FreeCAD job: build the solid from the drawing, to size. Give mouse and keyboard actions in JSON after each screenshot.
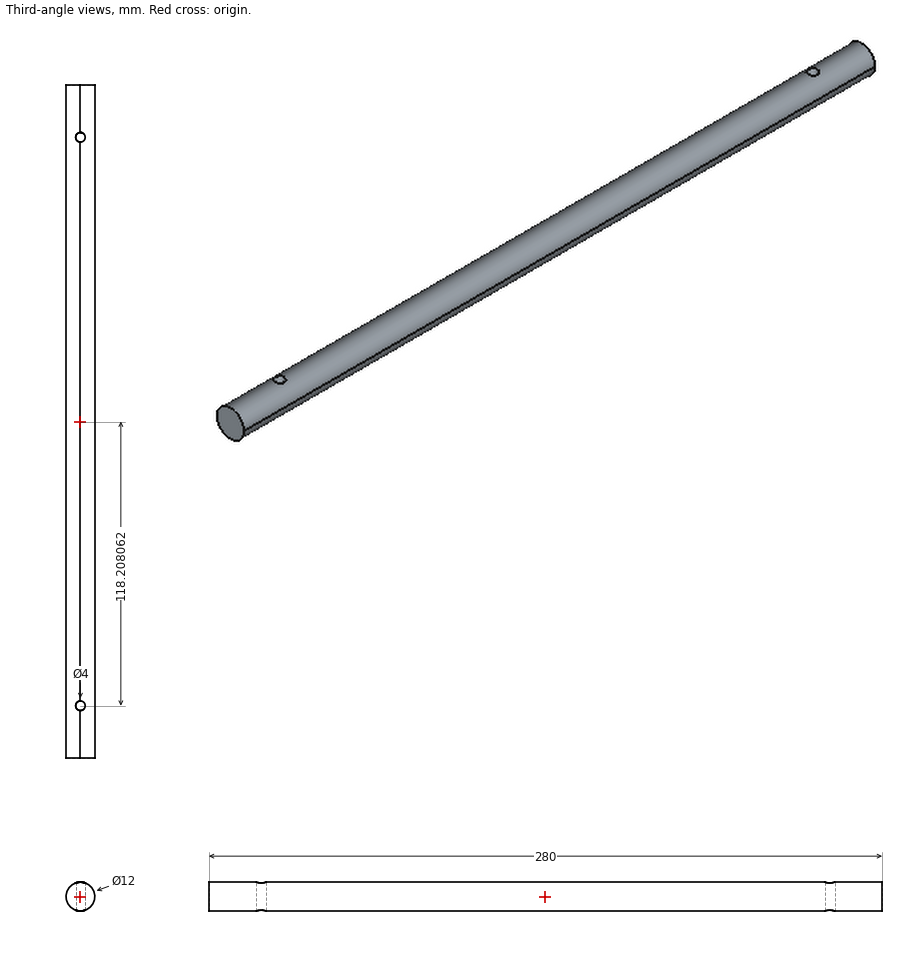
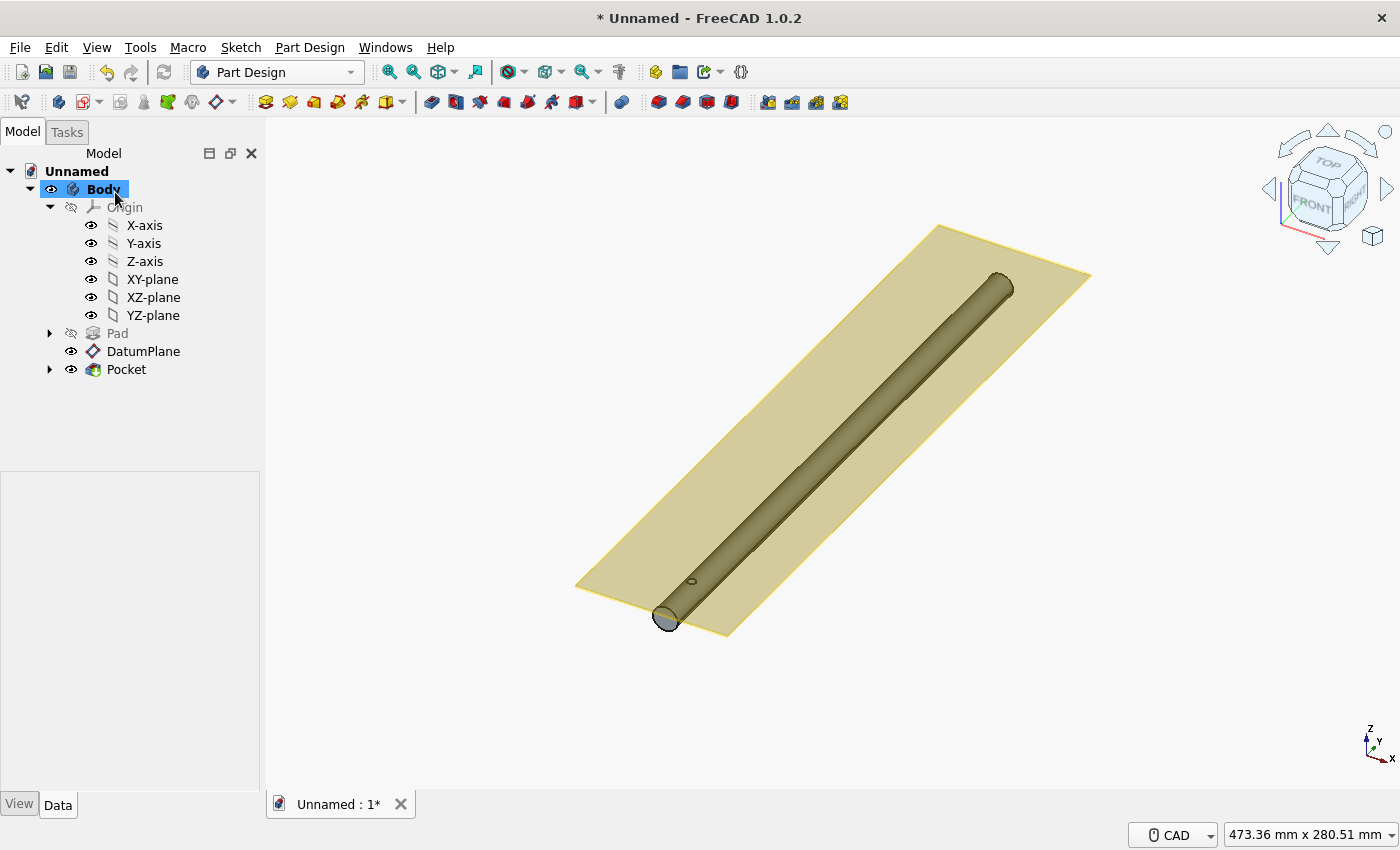
{"action": "left_click", "coordinate": [116, 351]}
{"action": "key", "text": "space"}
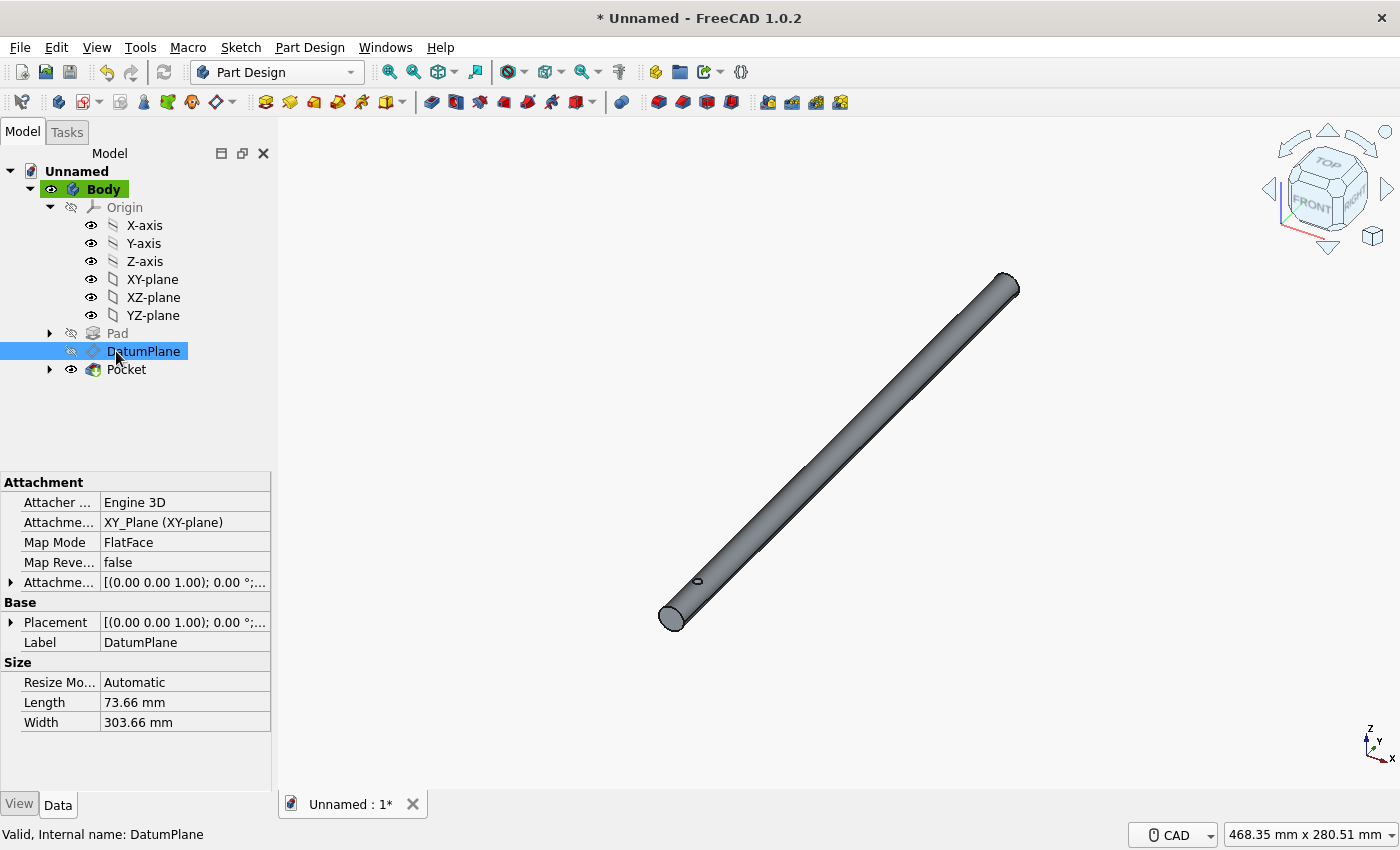
{"action": "left_click", "coordinate": [116, 369]}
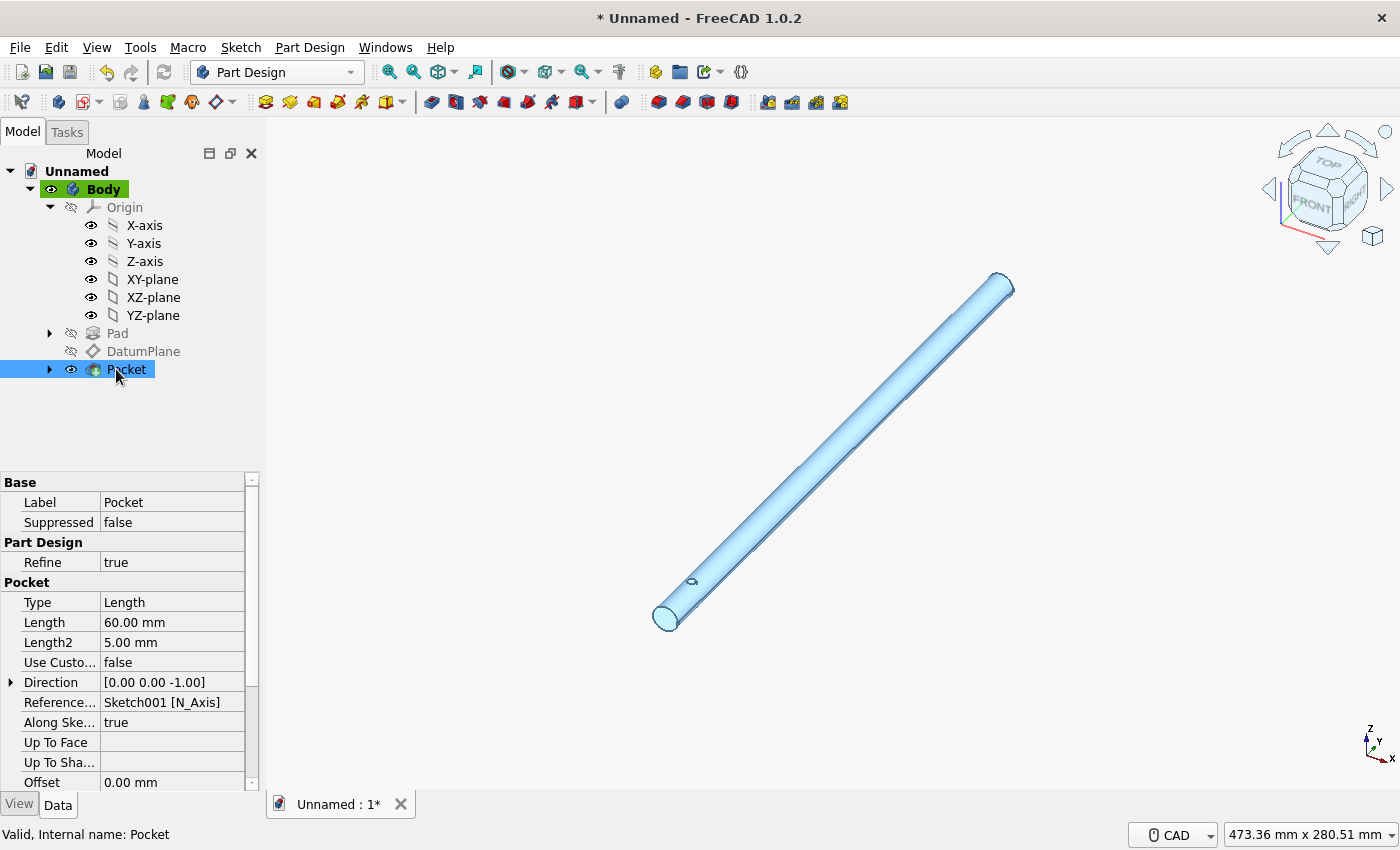
{"action": "left_click", "coordinate": [768, 102]}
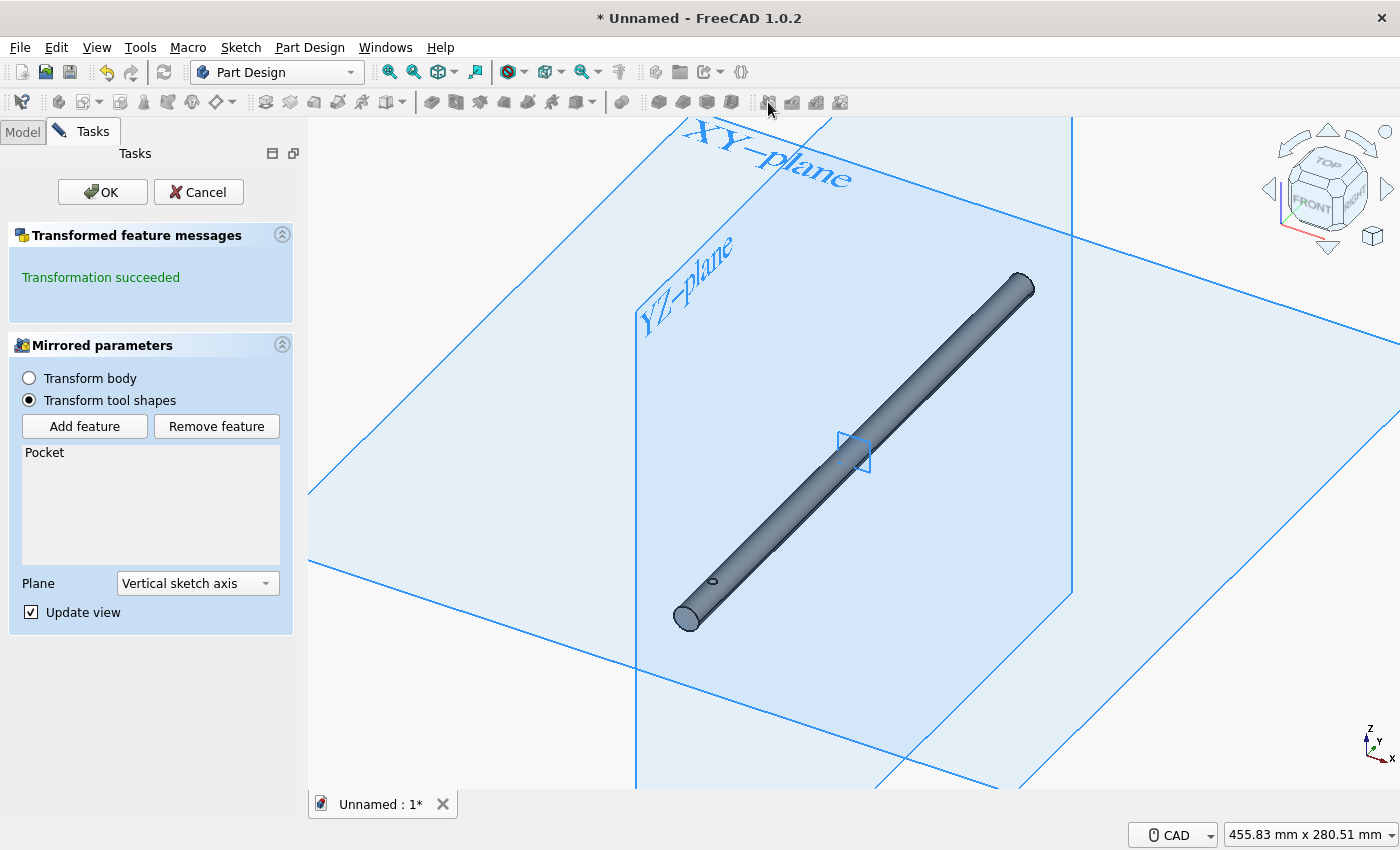
{"action": "left_click", "coordinate": [198, 584]}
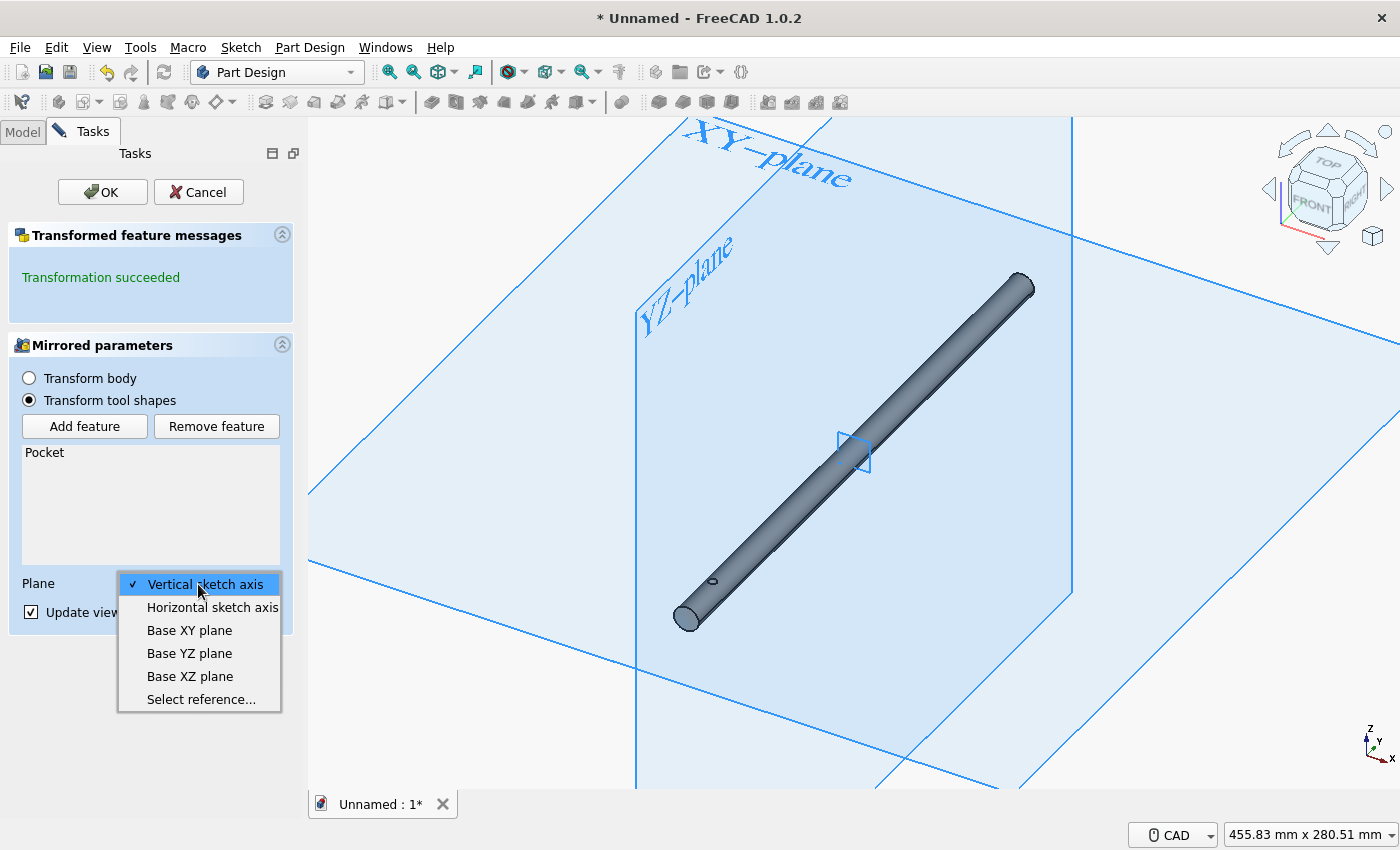
{"action": "left_click", "coordinate": [198, 676]}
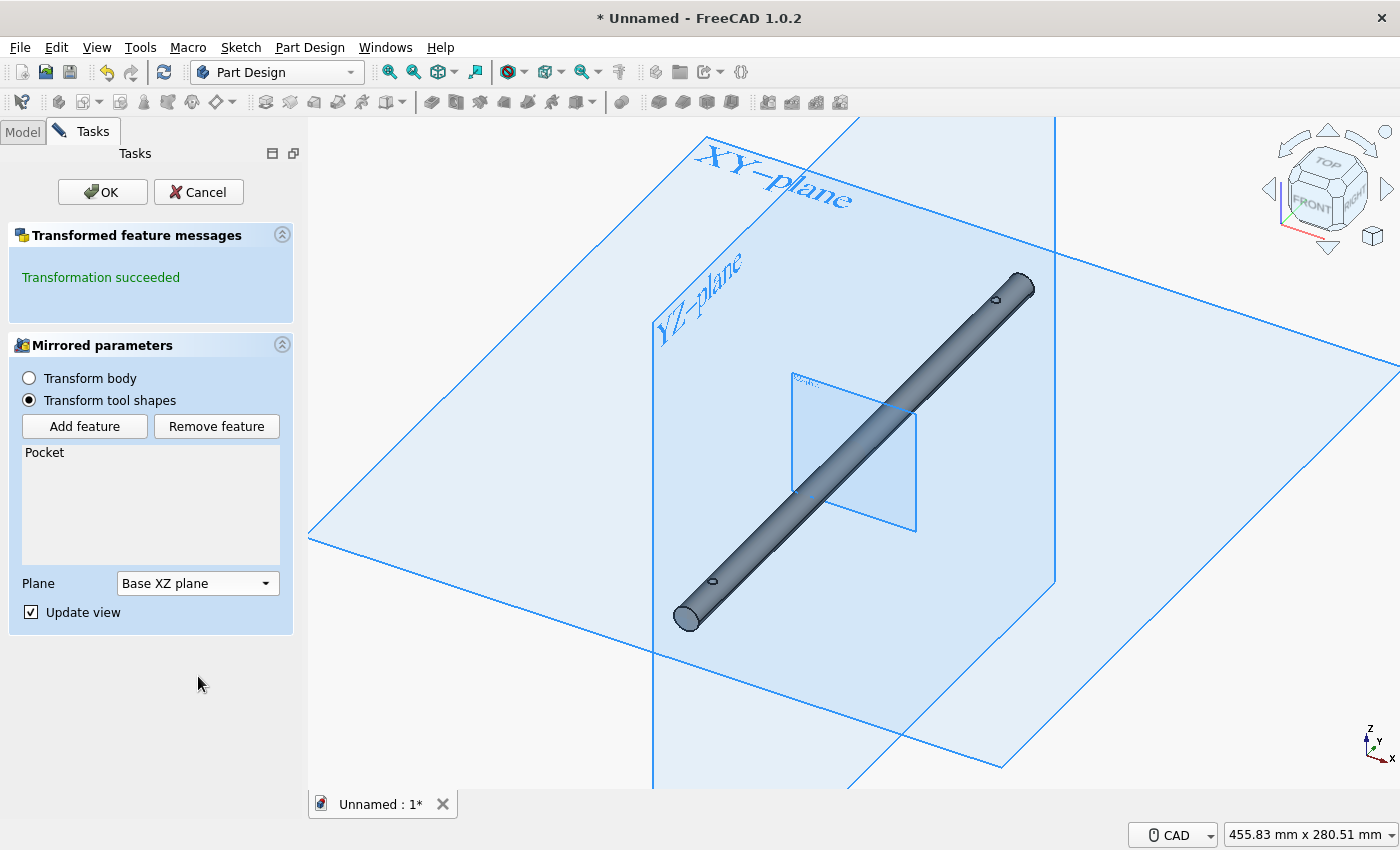
{"action": "left_click", "coordinate": [103, 192]}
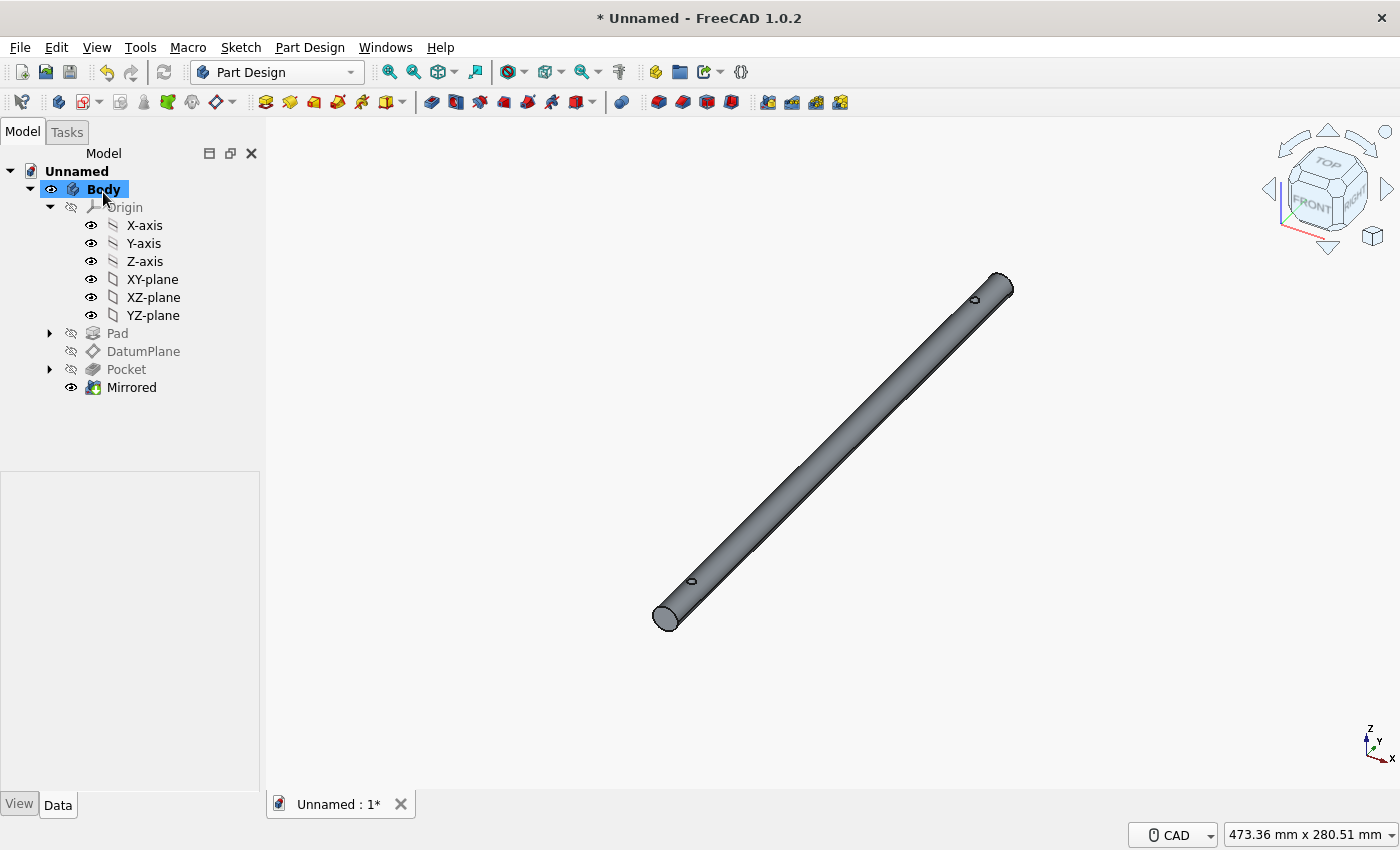
{"action": "key", "text": "0"}